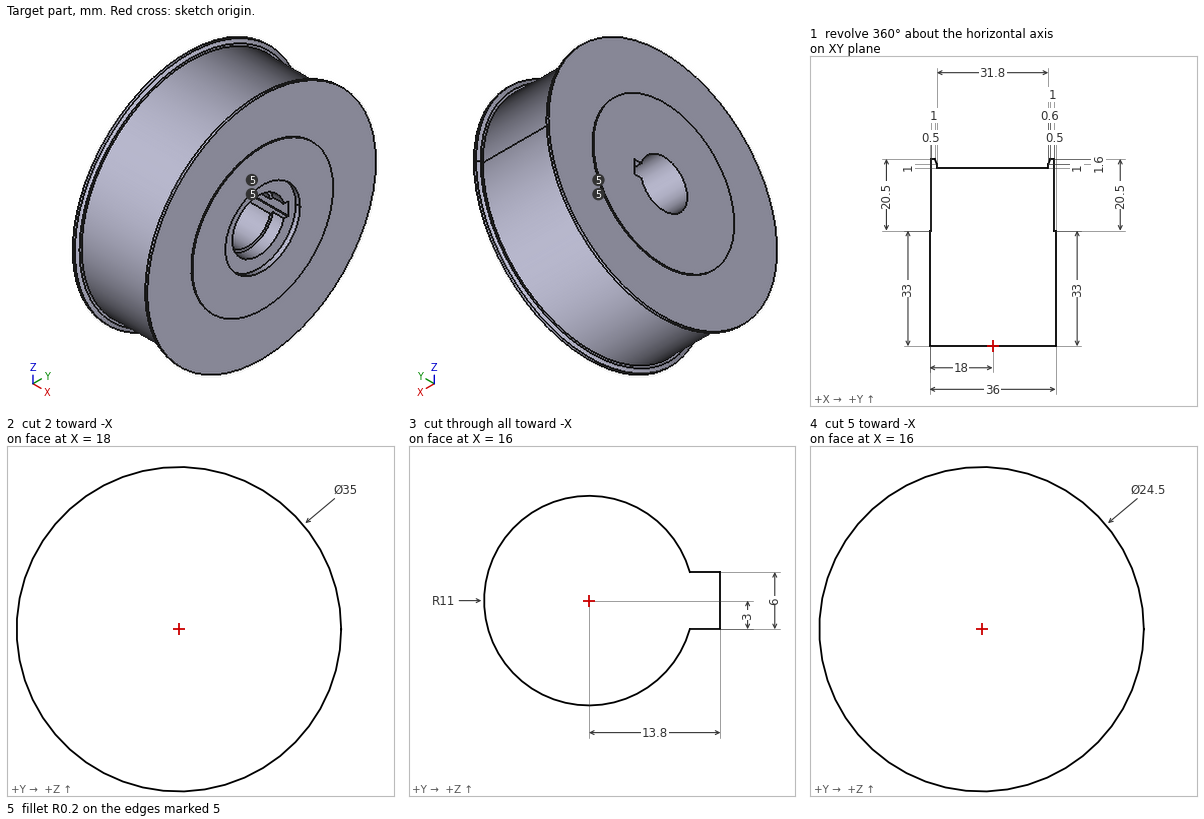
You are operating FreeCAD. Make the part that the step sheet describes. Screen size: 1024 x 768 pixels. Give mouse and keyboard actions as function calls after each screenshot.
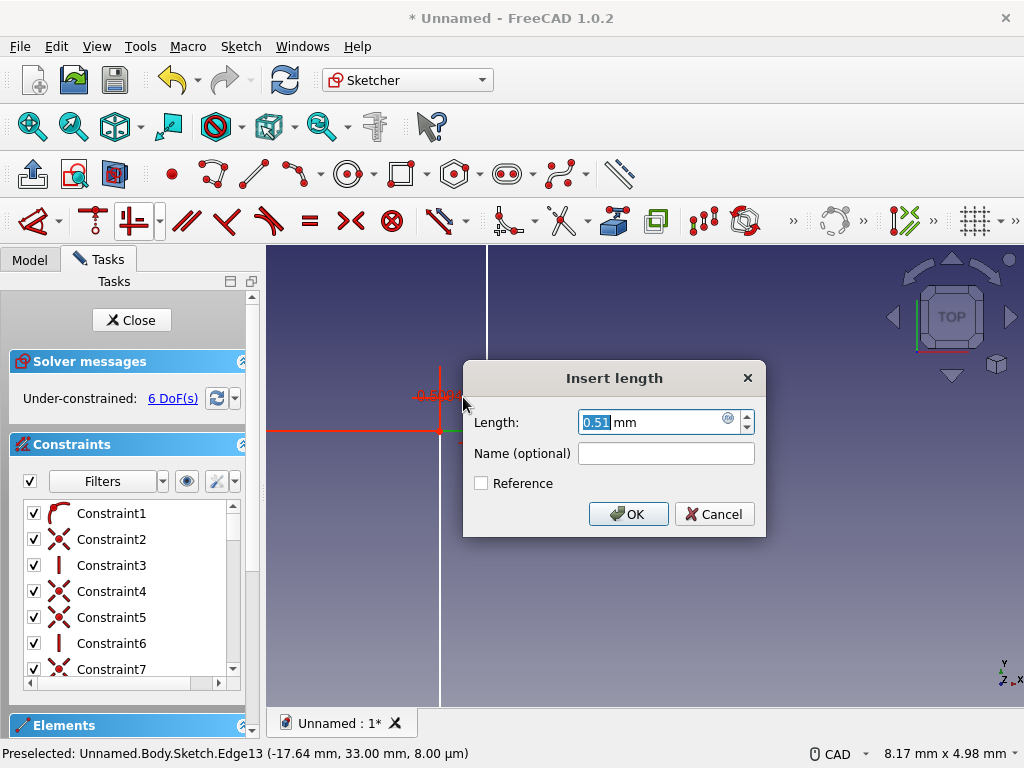
text(0.5)
key(Return)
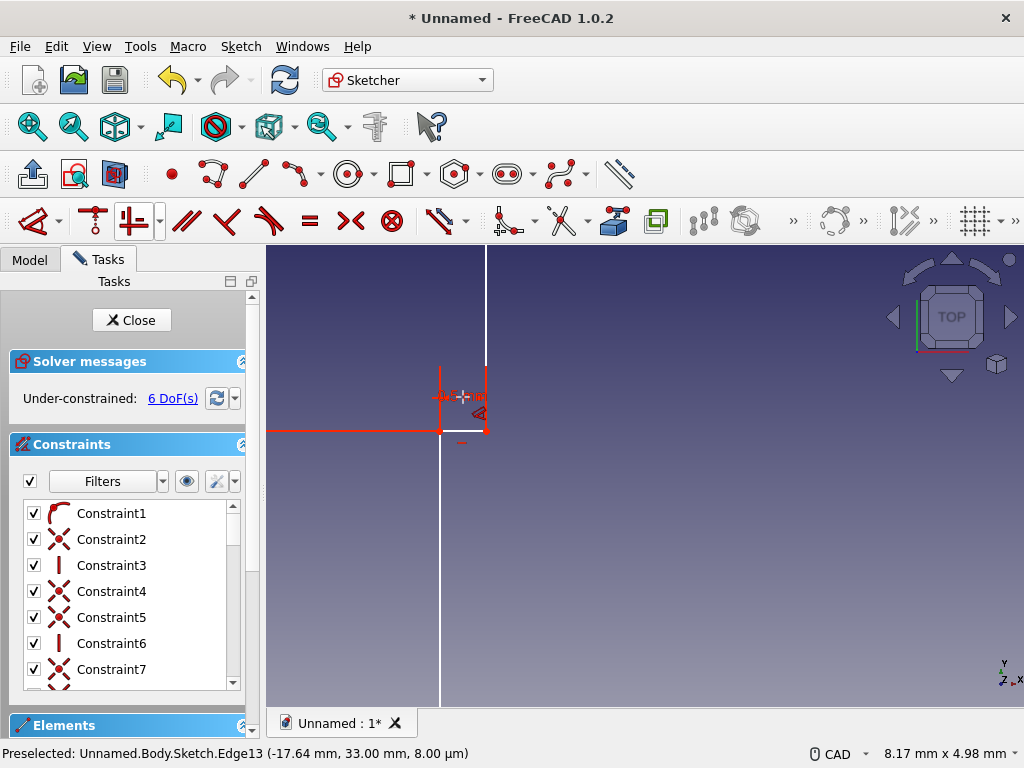
scroll(477, 441, down, 14)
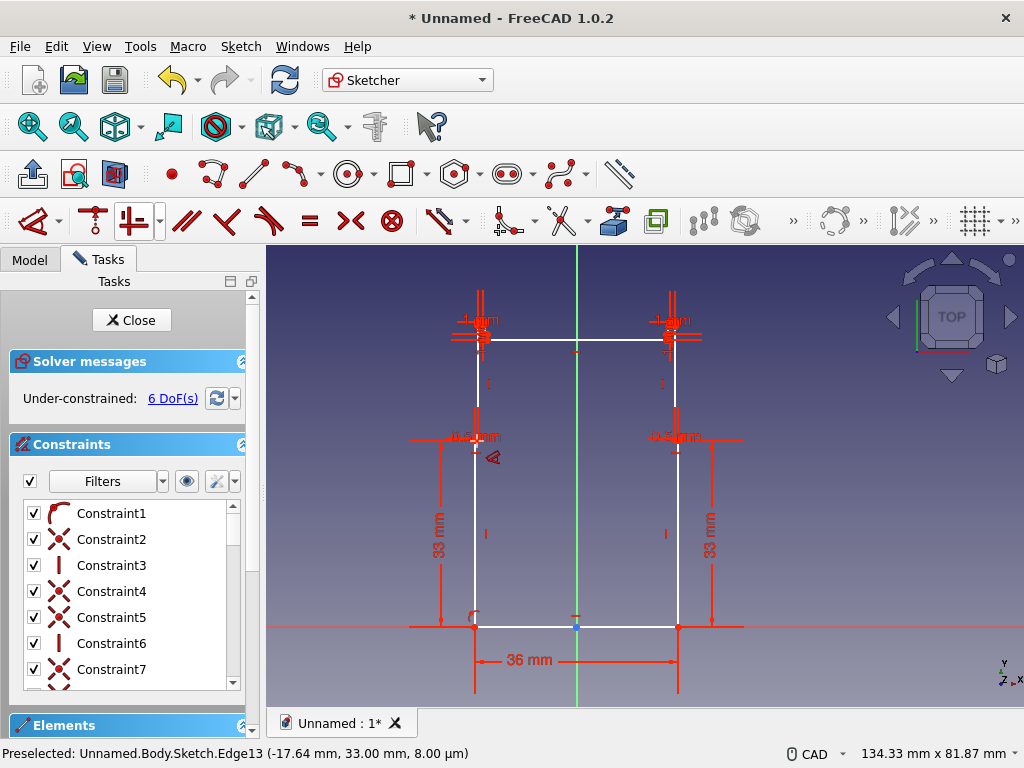
click(475, 627)
click(526, 593)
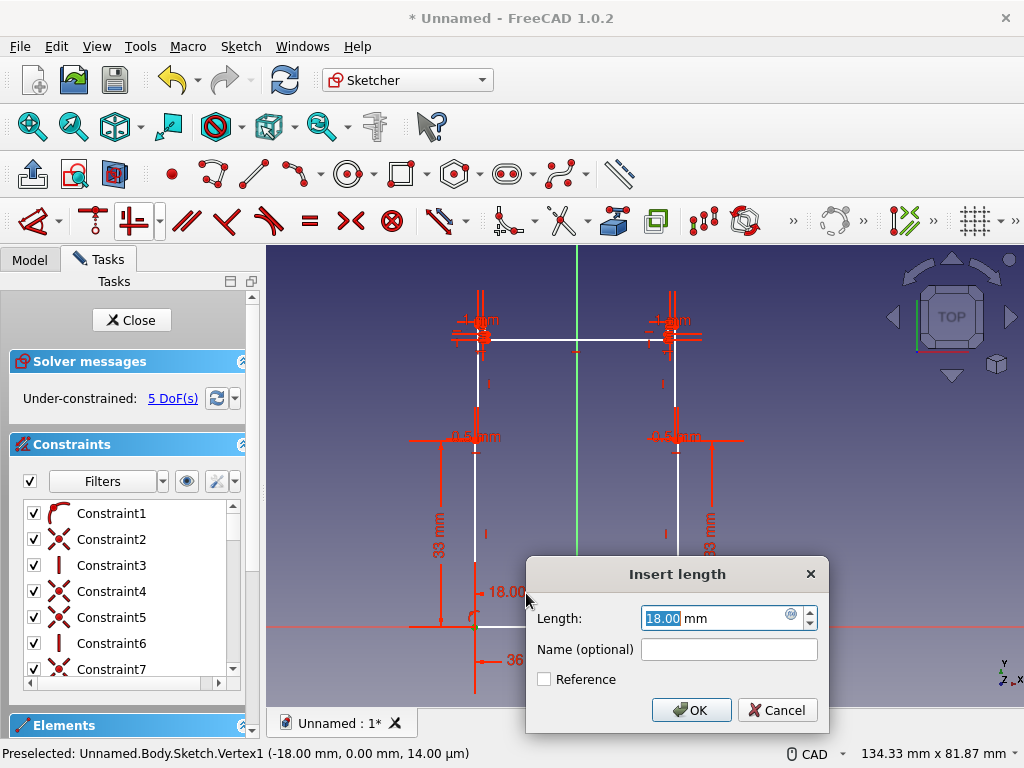
text(18)
key(Return)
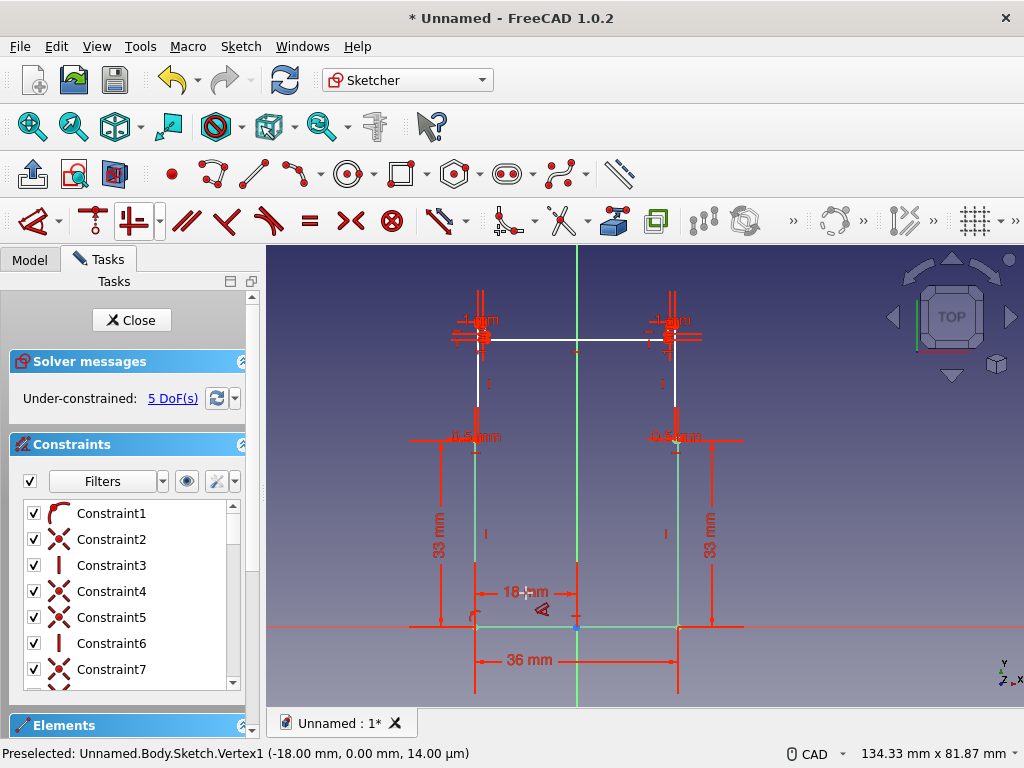
click(675, 406)
click(709, 383)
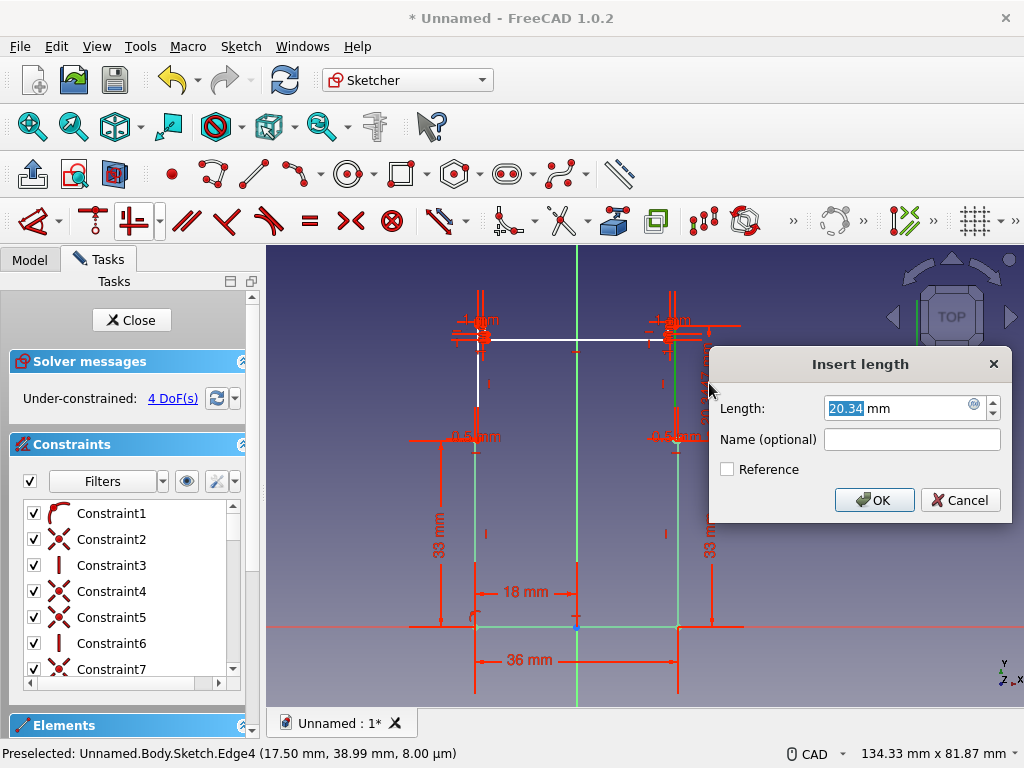
text(20.5)
key(Return)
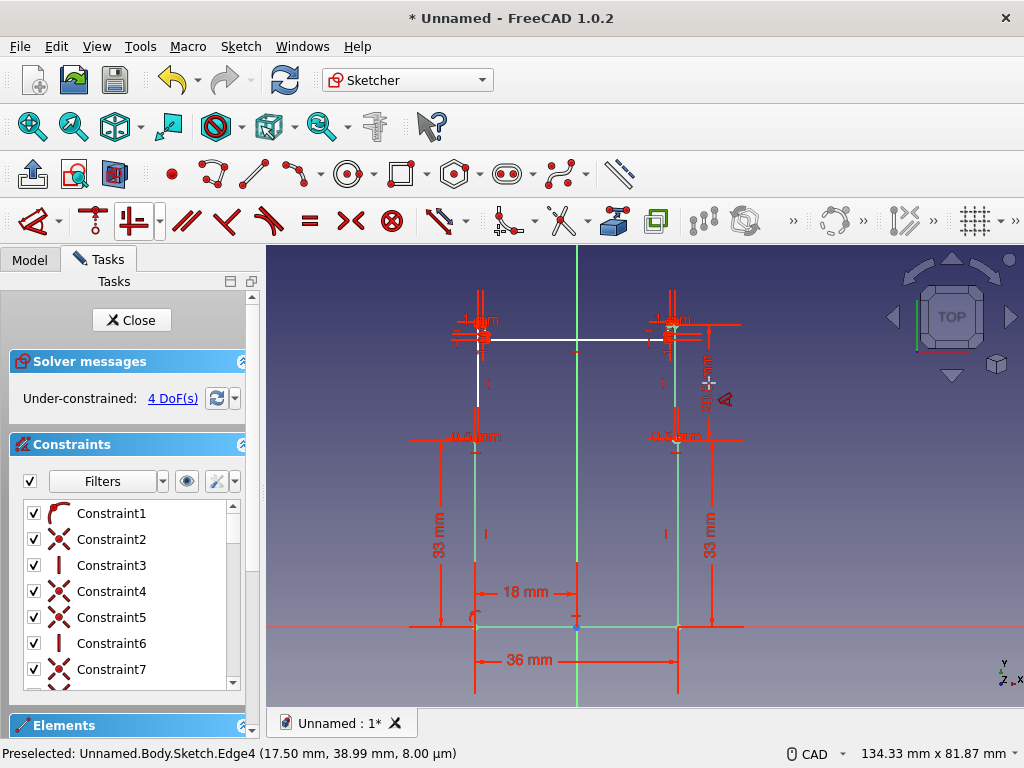
click(613, 340)
click(535, 374)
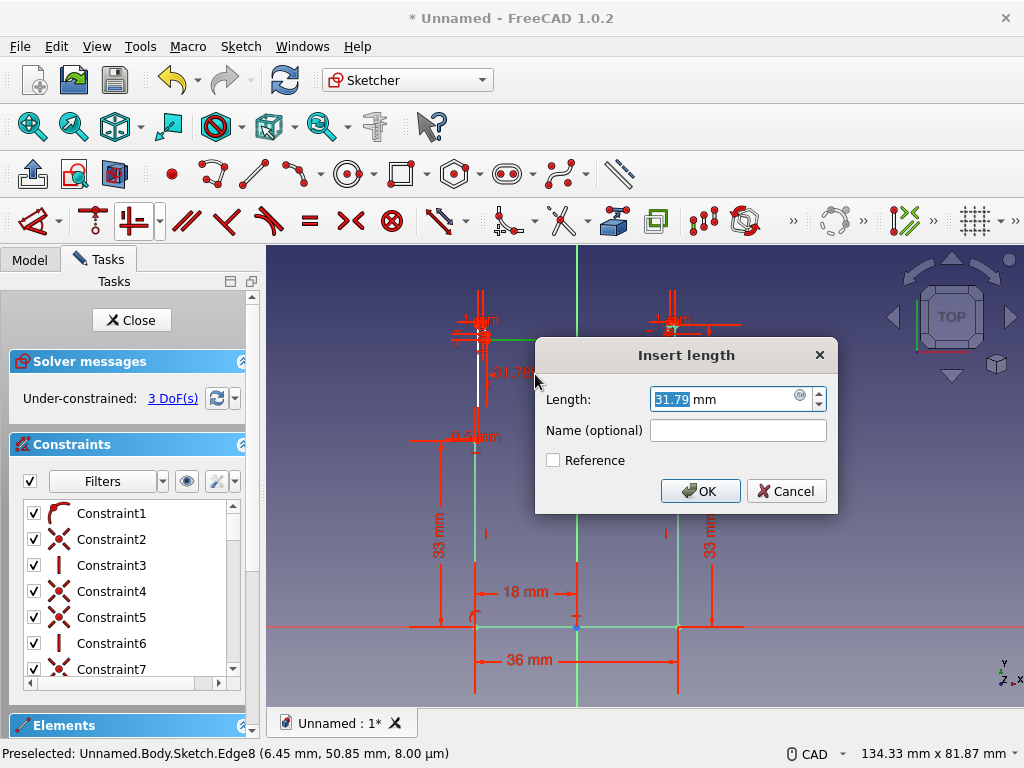
text(31.8)
key(Return)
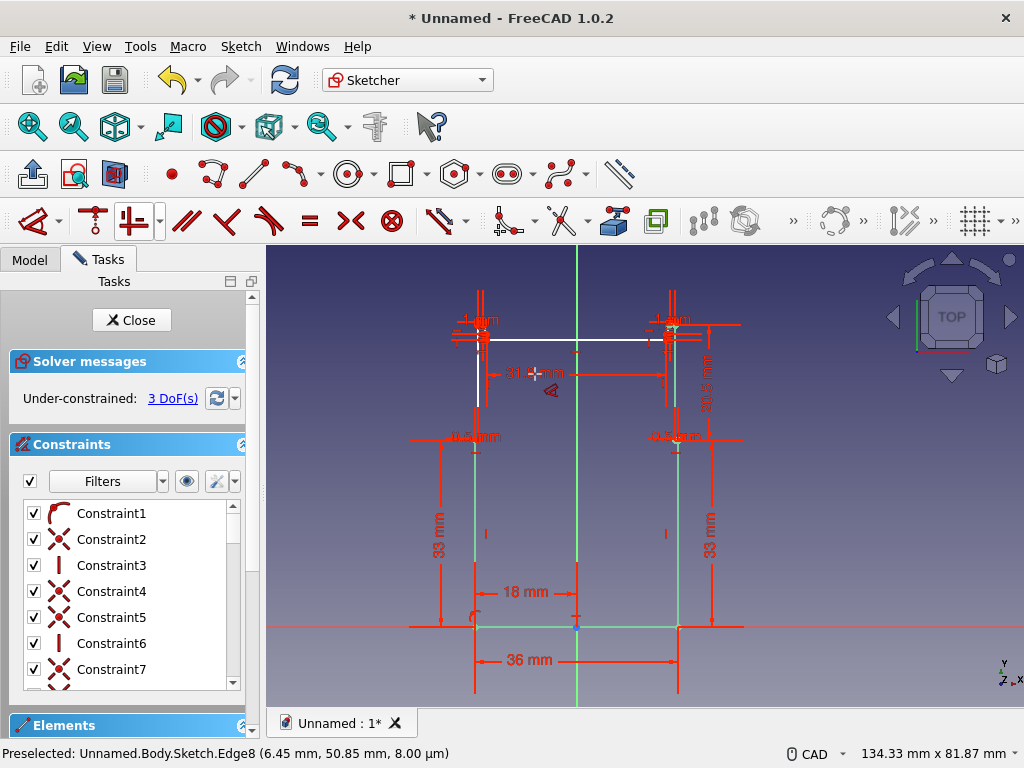
click(478, 360)
click(444, 383)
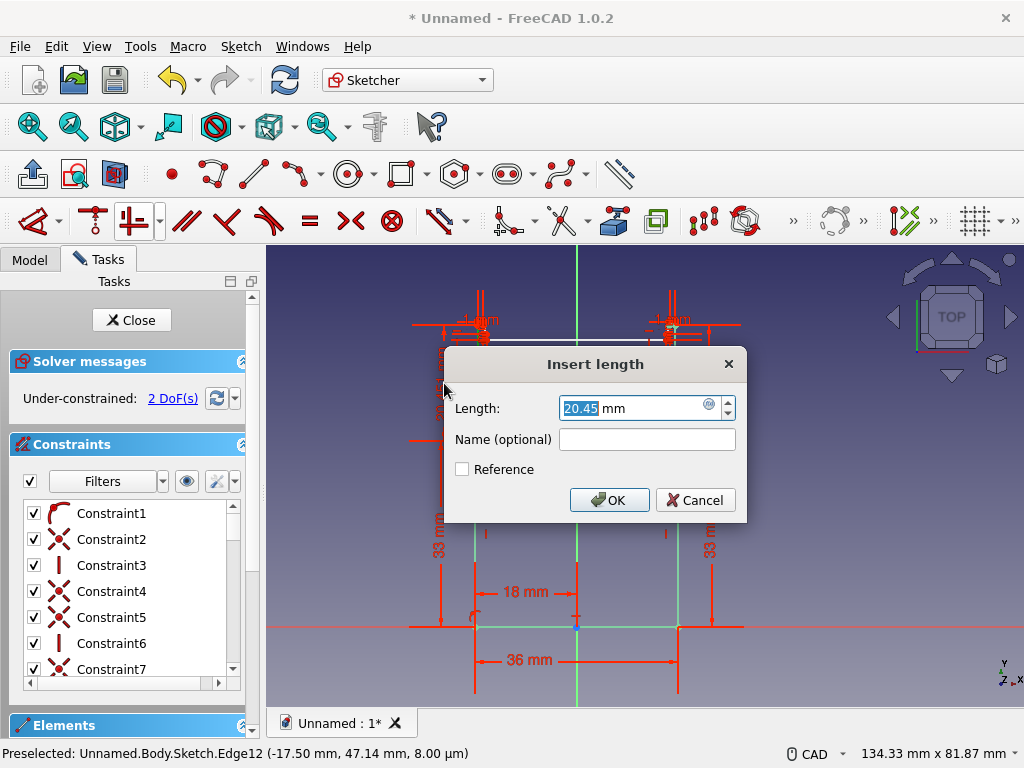
text(20.5)
key(Return)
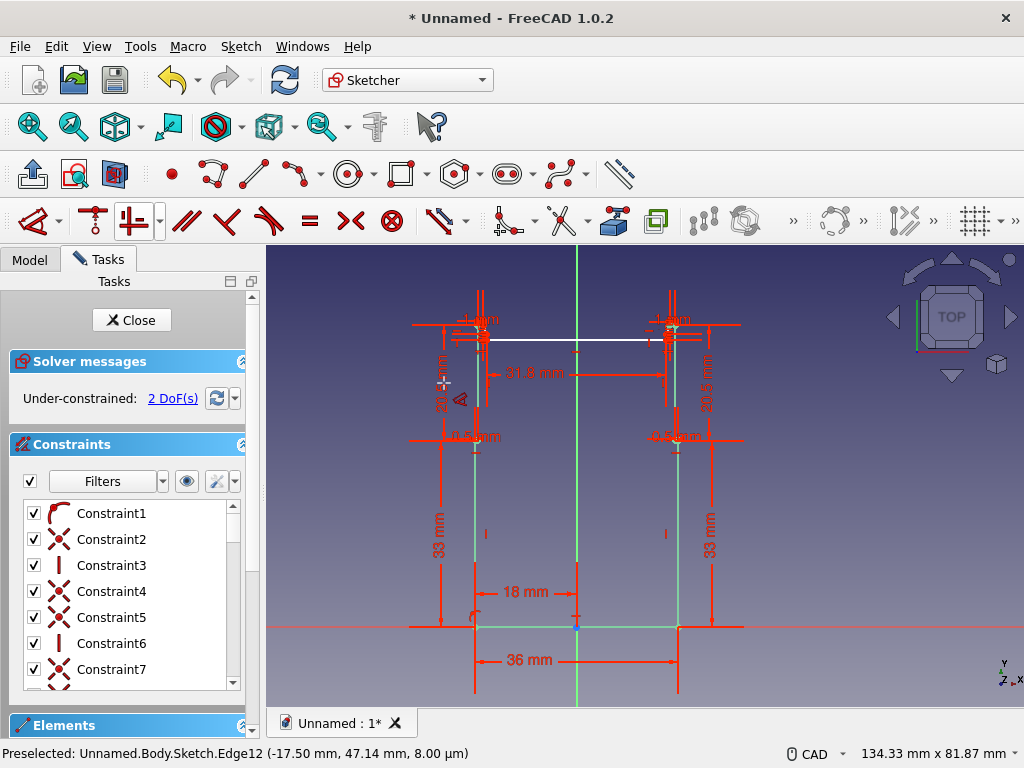
scroll(668, 330, up, 13)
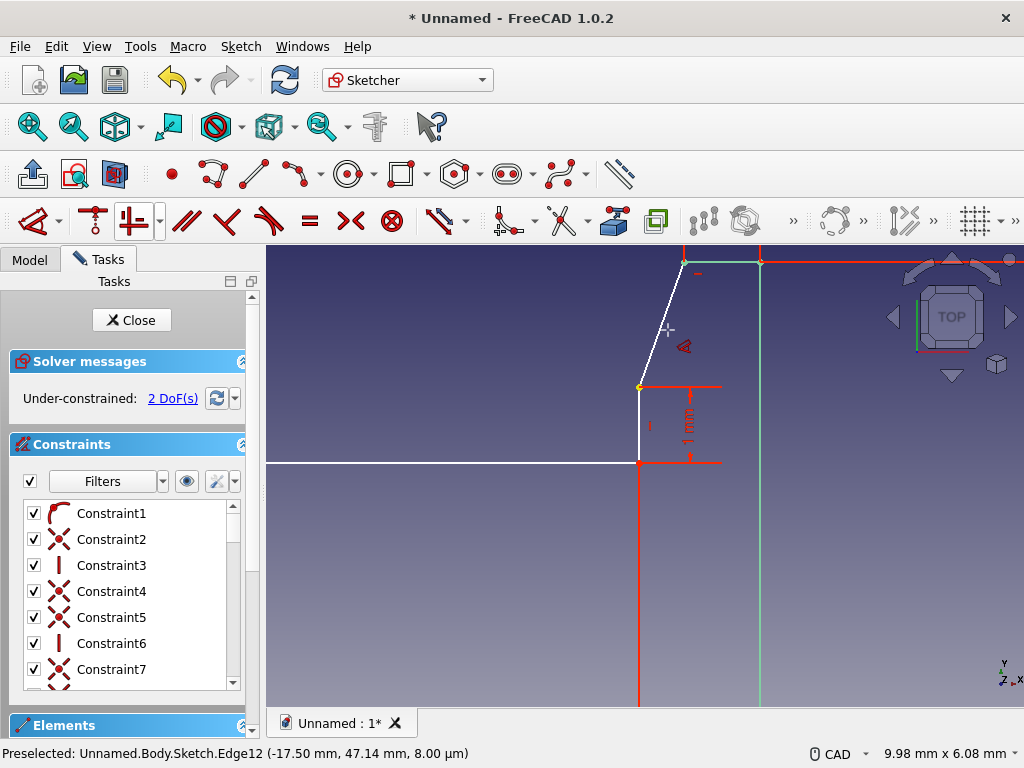
click(662, 325)
click(662, 469)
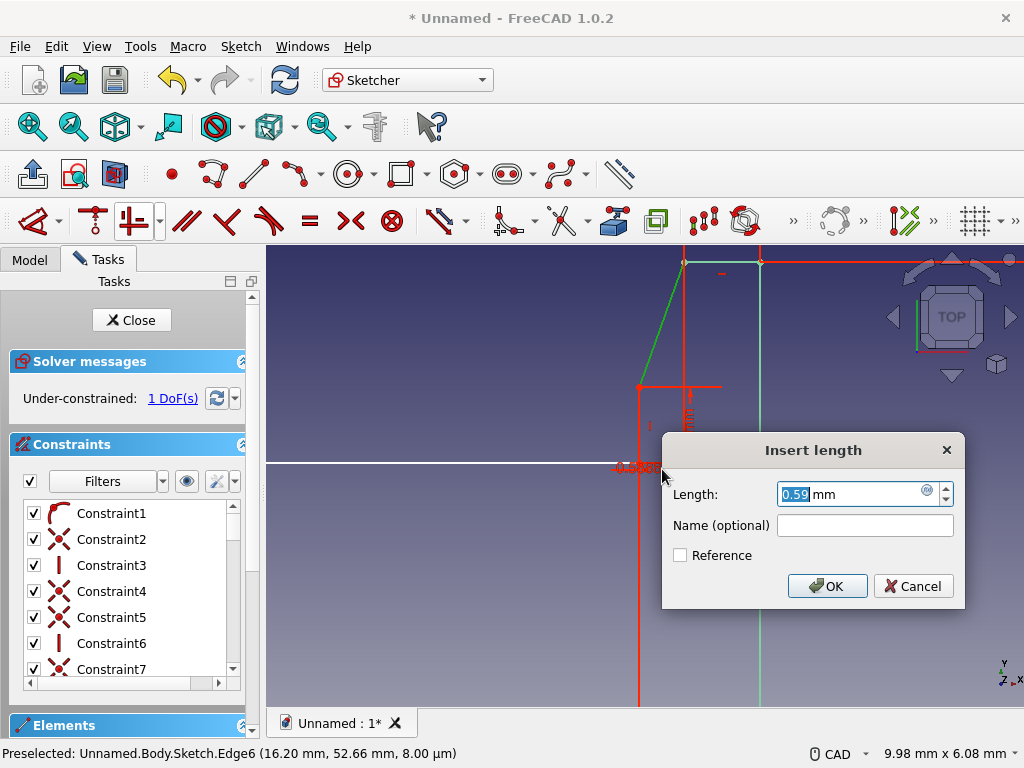
text(0.6)
key(Return)